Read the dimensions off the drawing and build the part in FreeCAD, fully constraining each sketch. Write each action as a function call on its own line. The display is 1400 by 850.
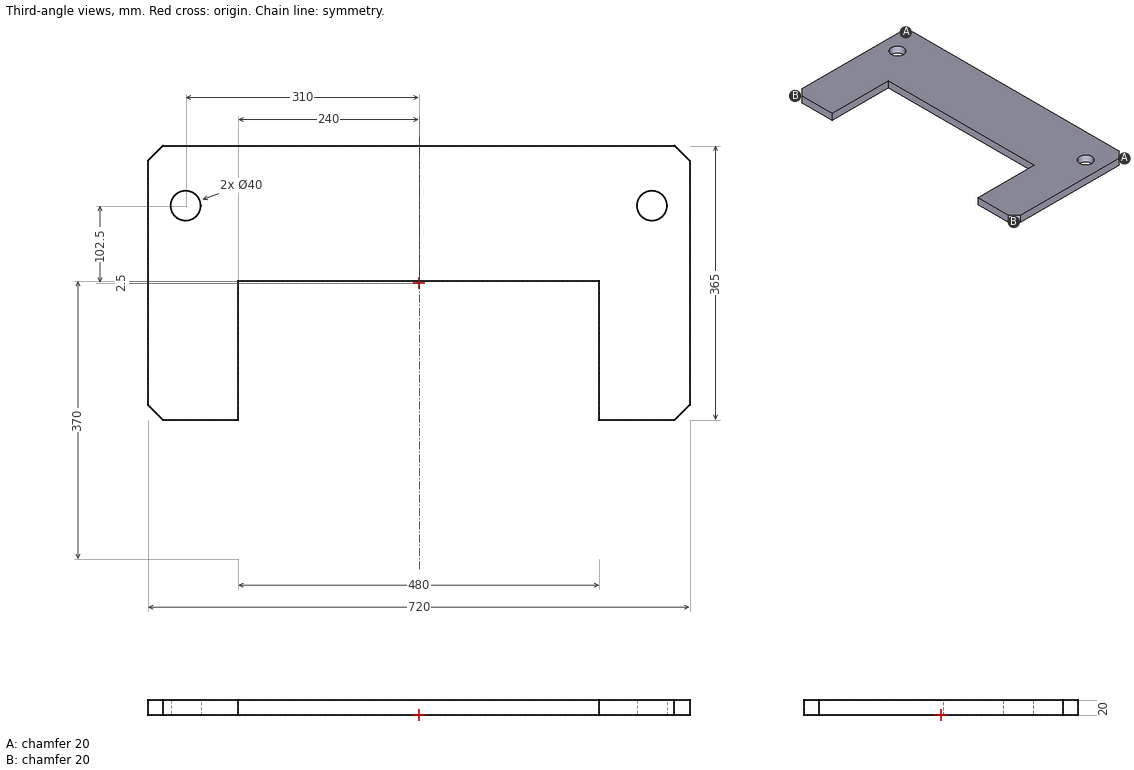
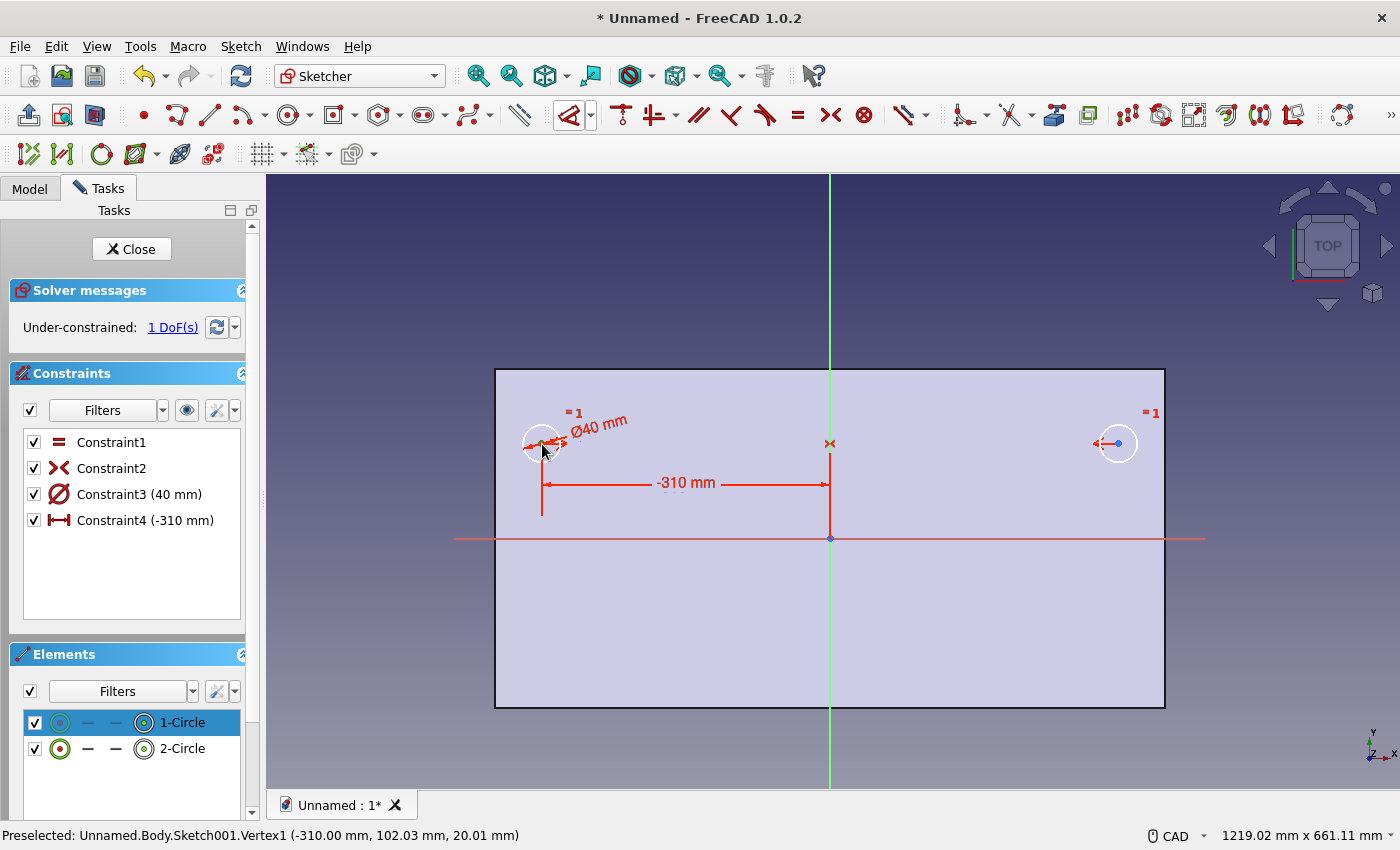
key(i)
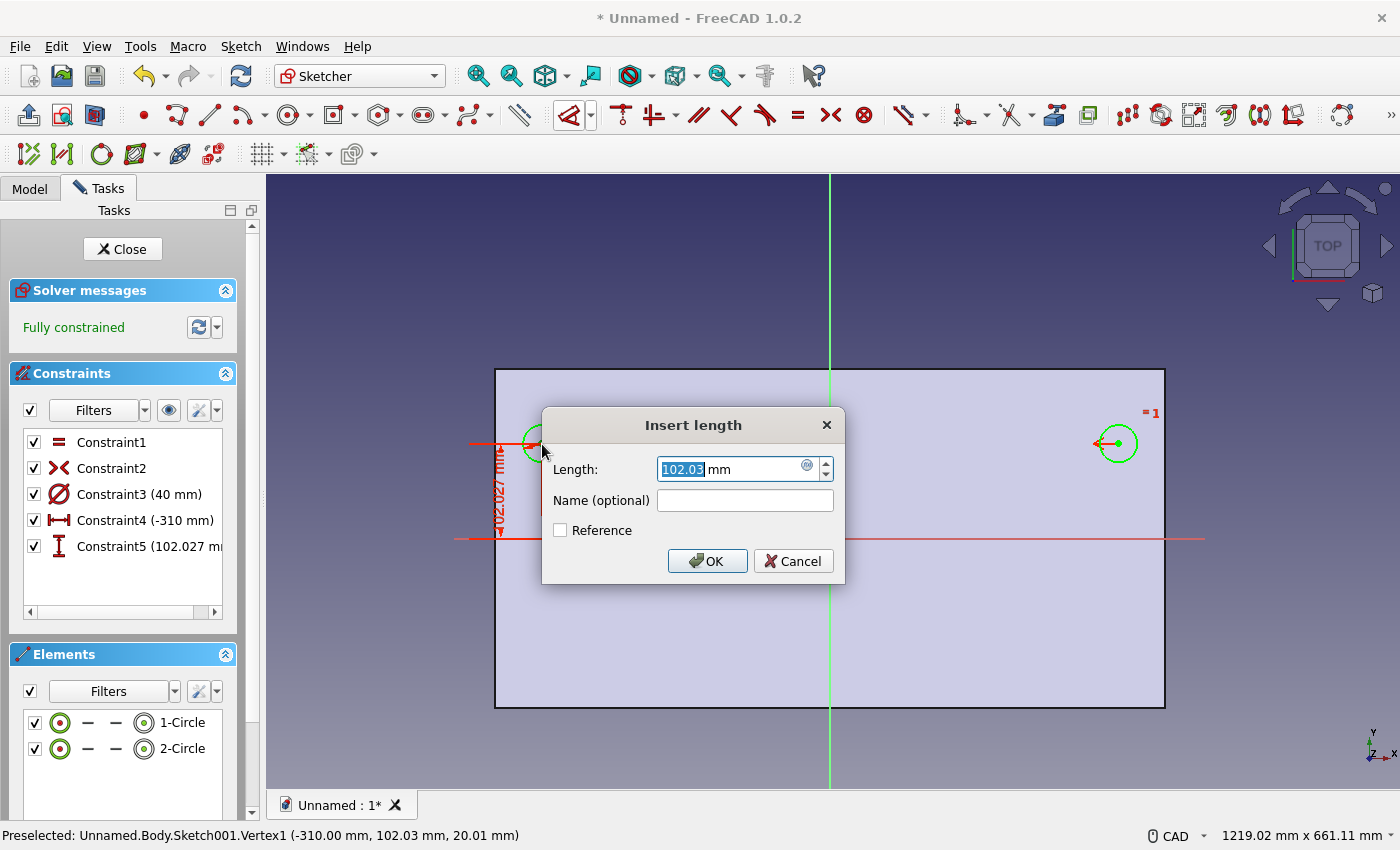
text(102.5)
key(Return)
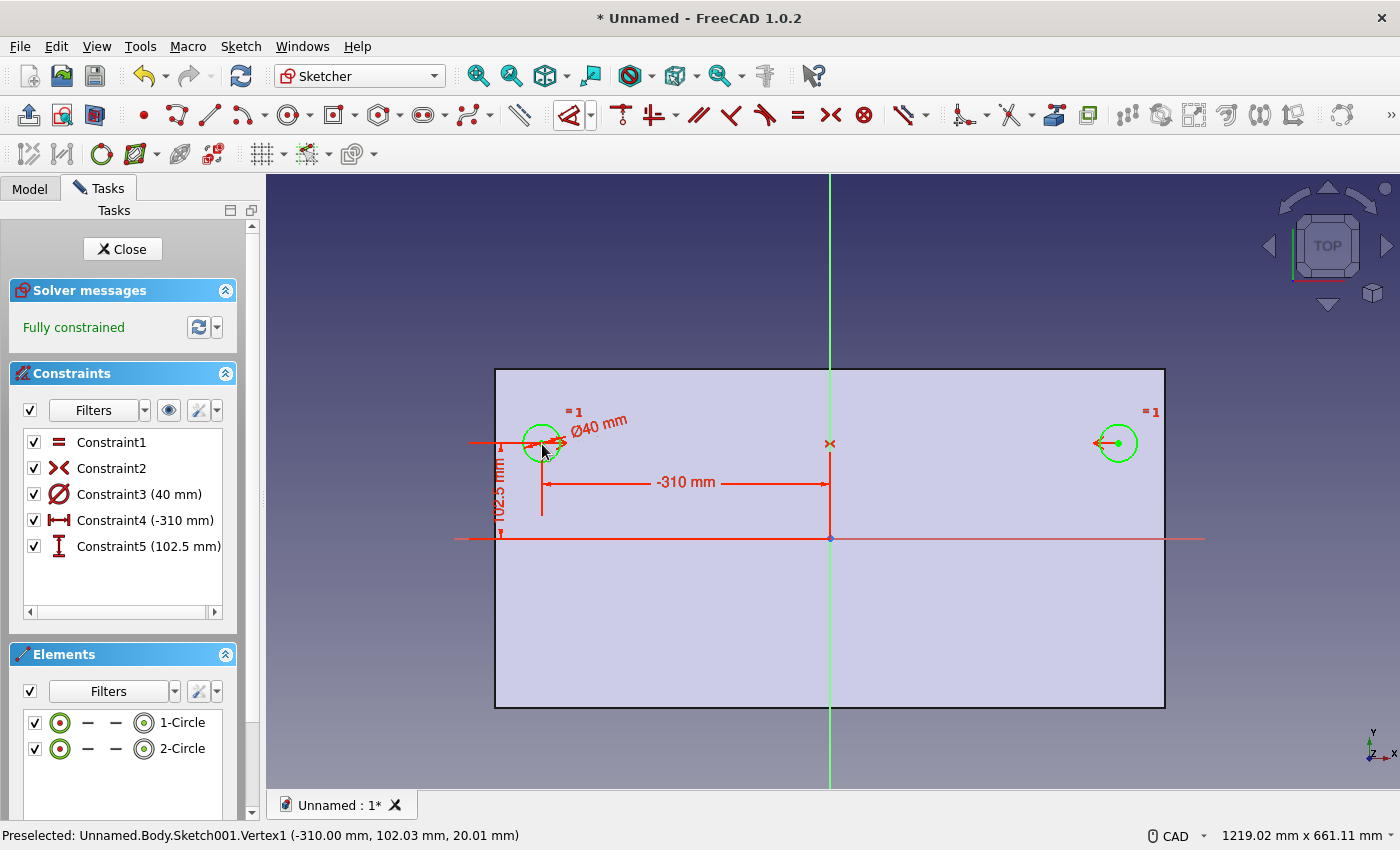
click(123, 249)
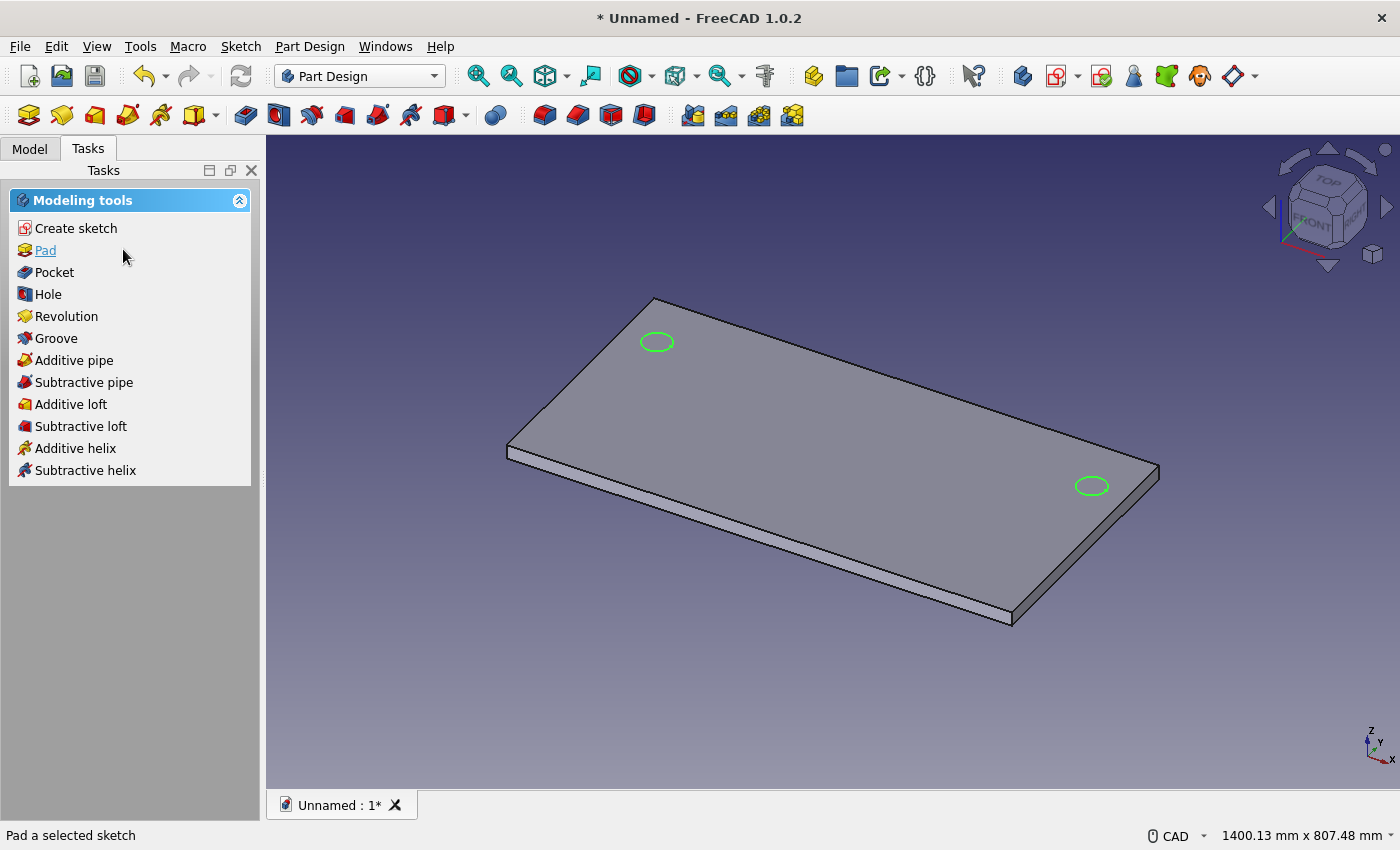
click(246, 116)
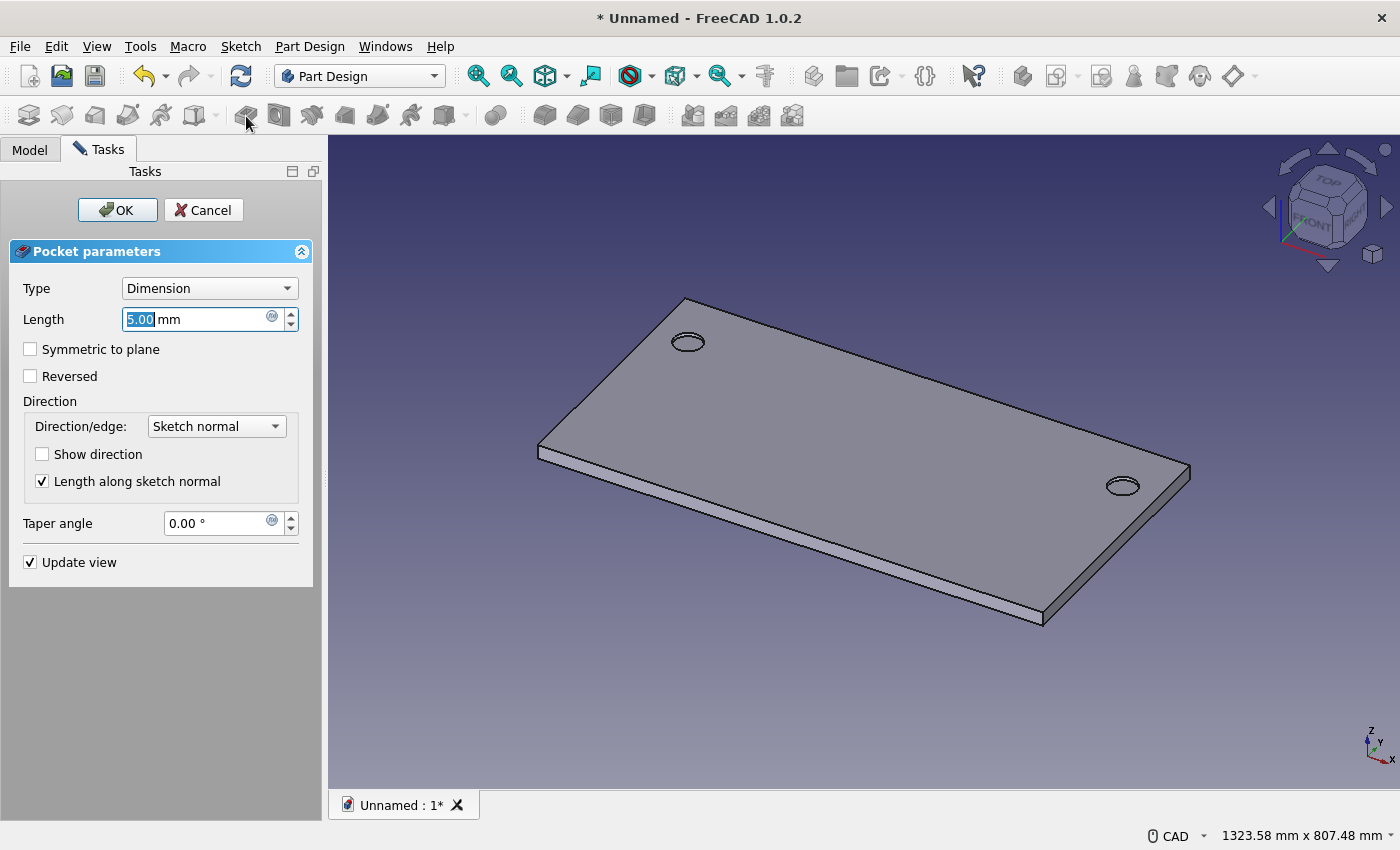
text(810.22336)
key(Tab)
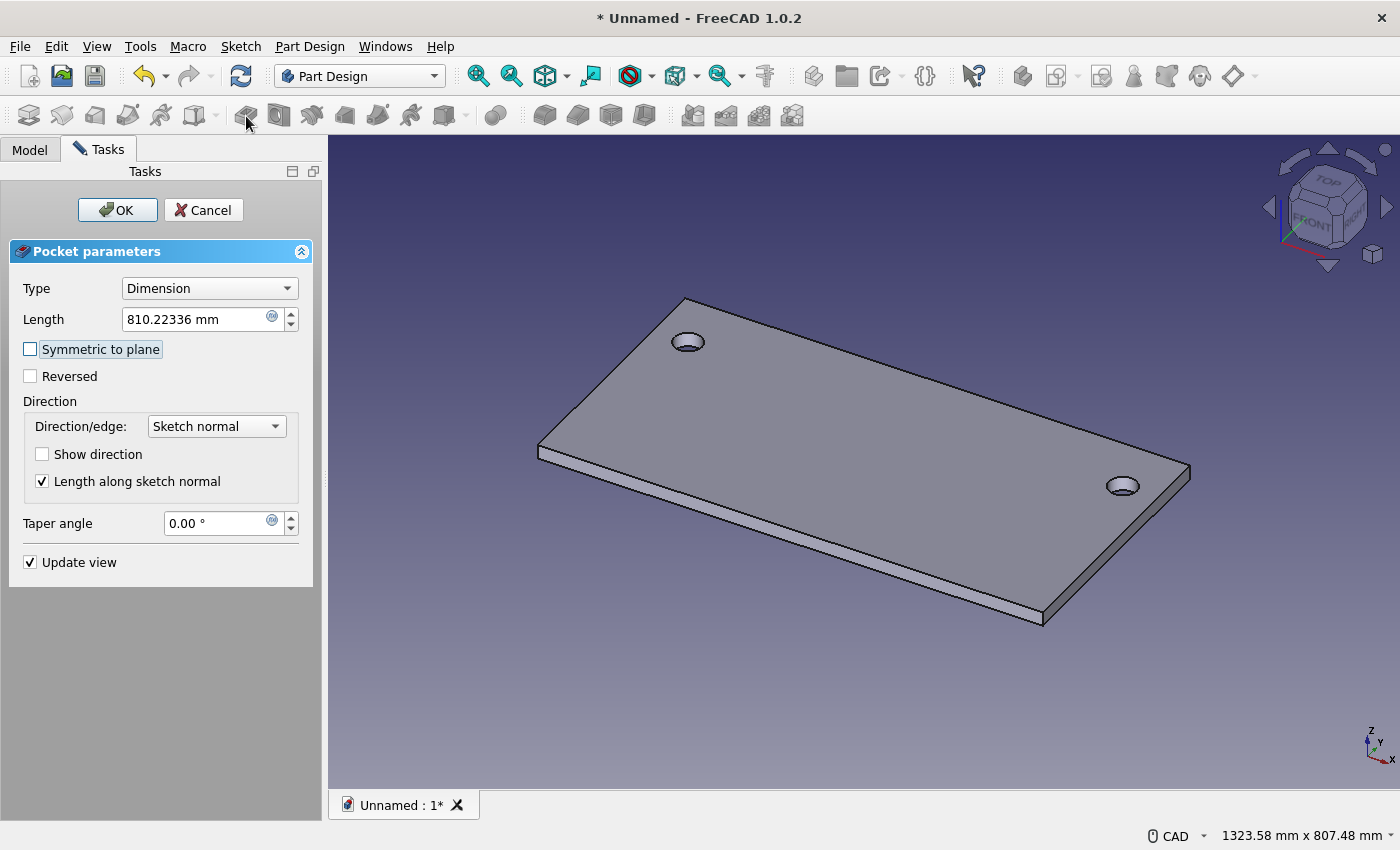
click(31, 349)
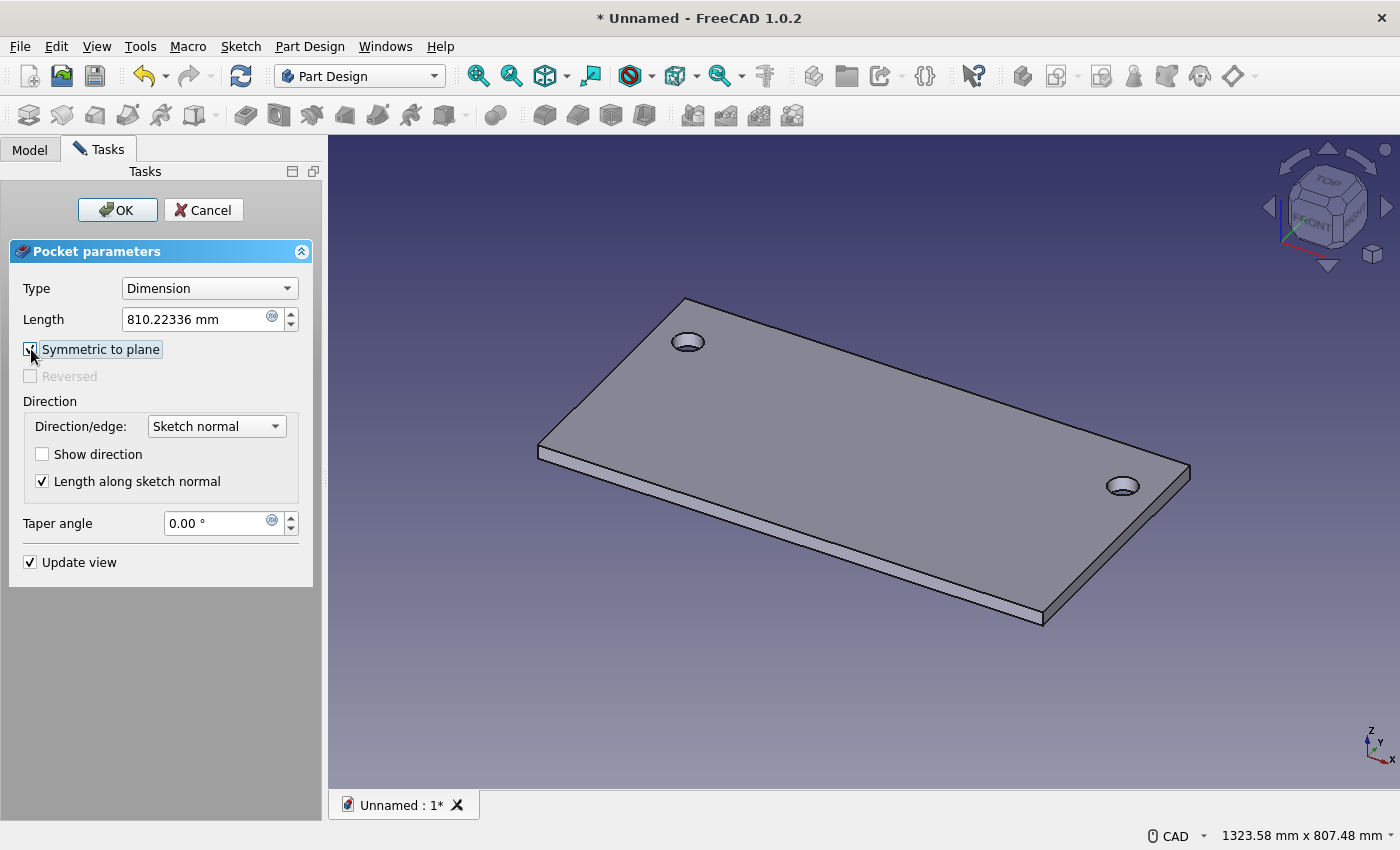
click(118, 210)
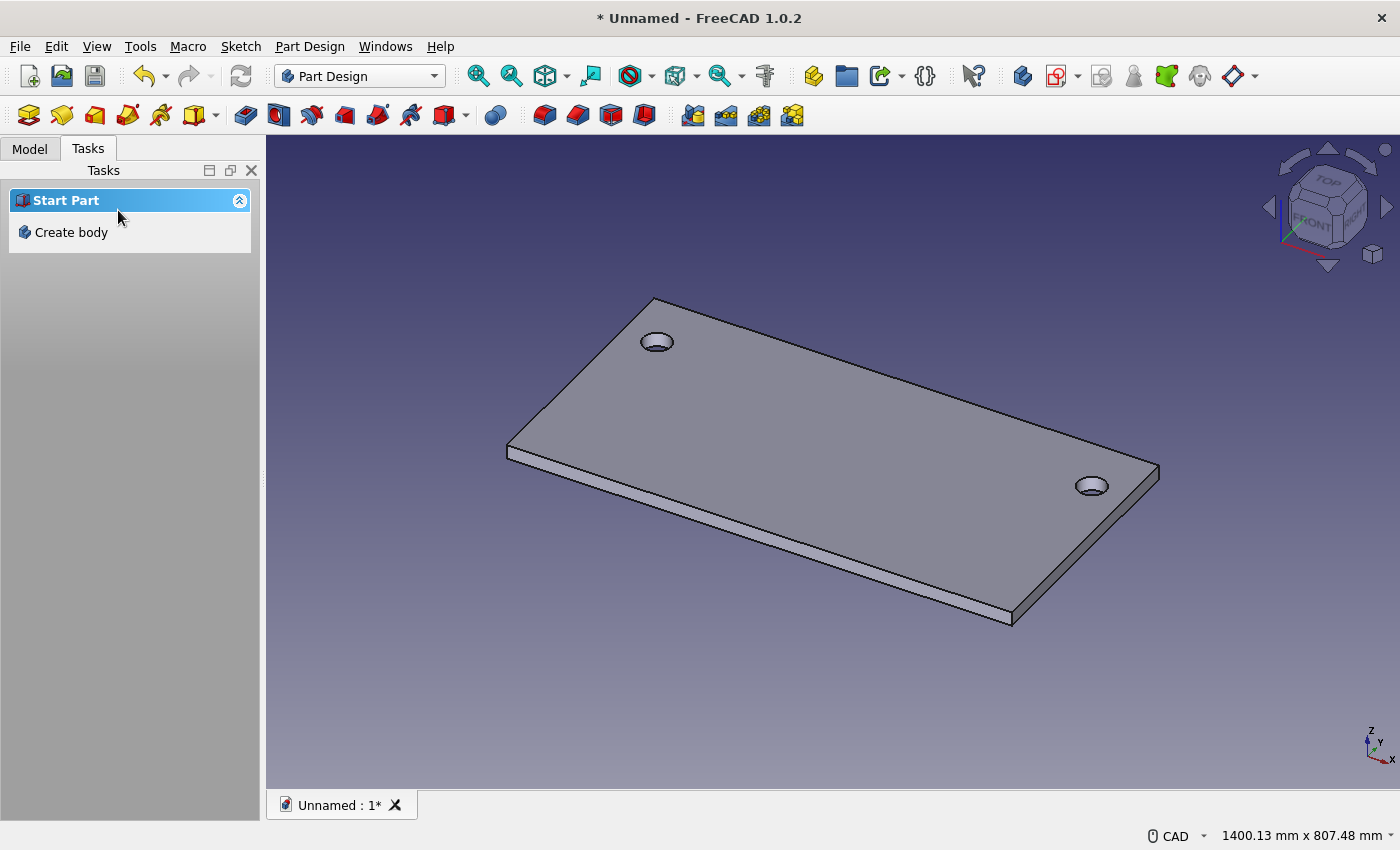
scroll(654, 304, up, 5)